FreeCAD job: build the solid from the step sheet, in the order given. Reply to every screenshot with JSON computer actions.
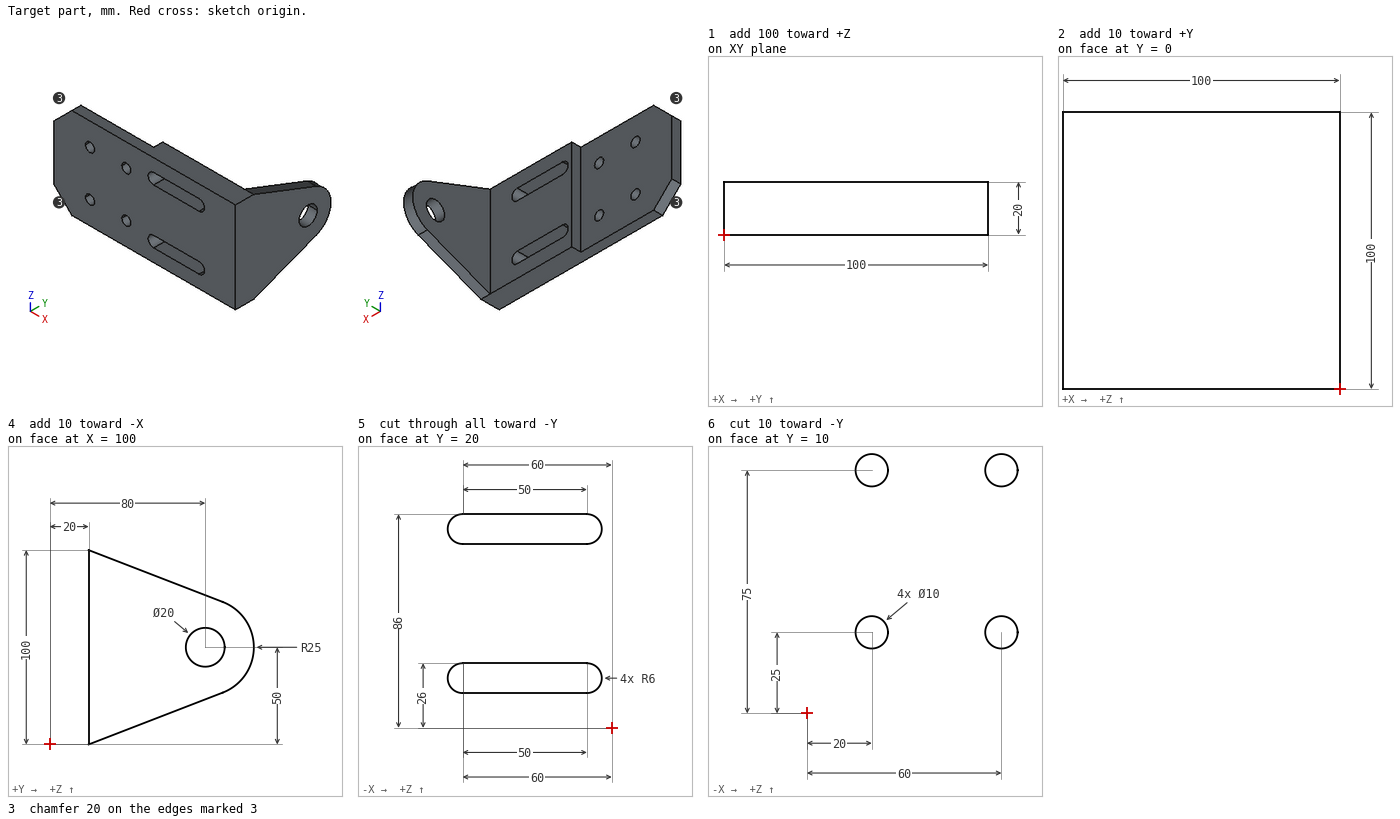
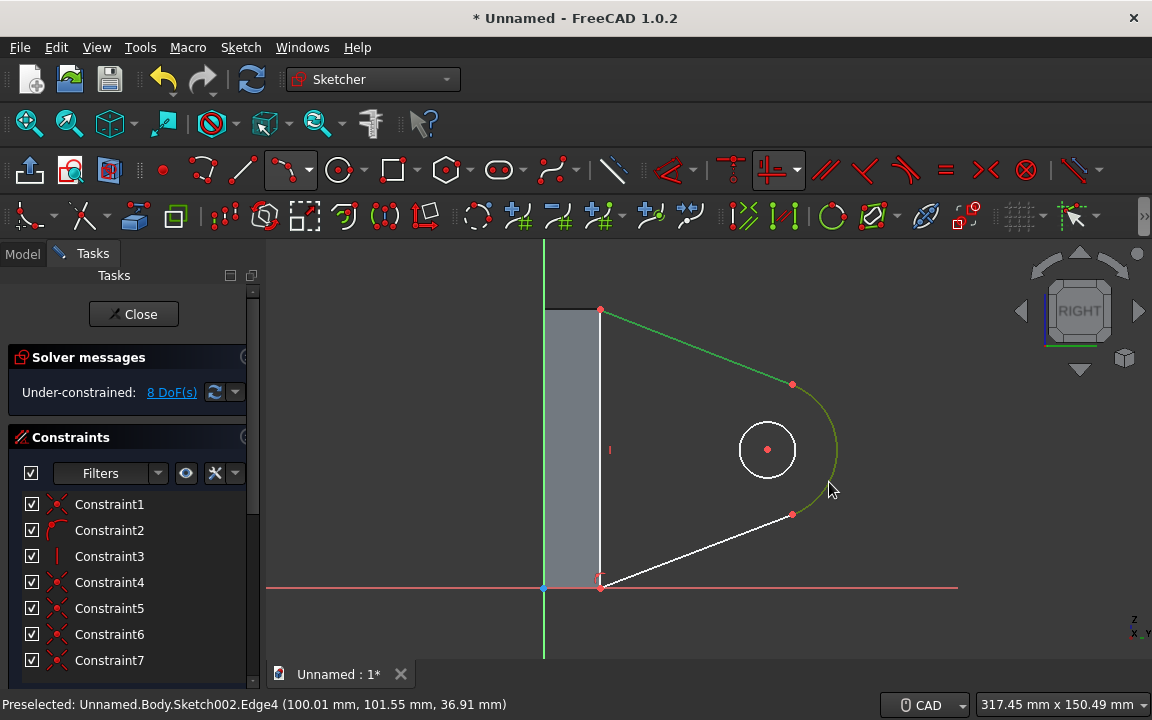
{"action": "left_click", "coordinate": [906, 170]}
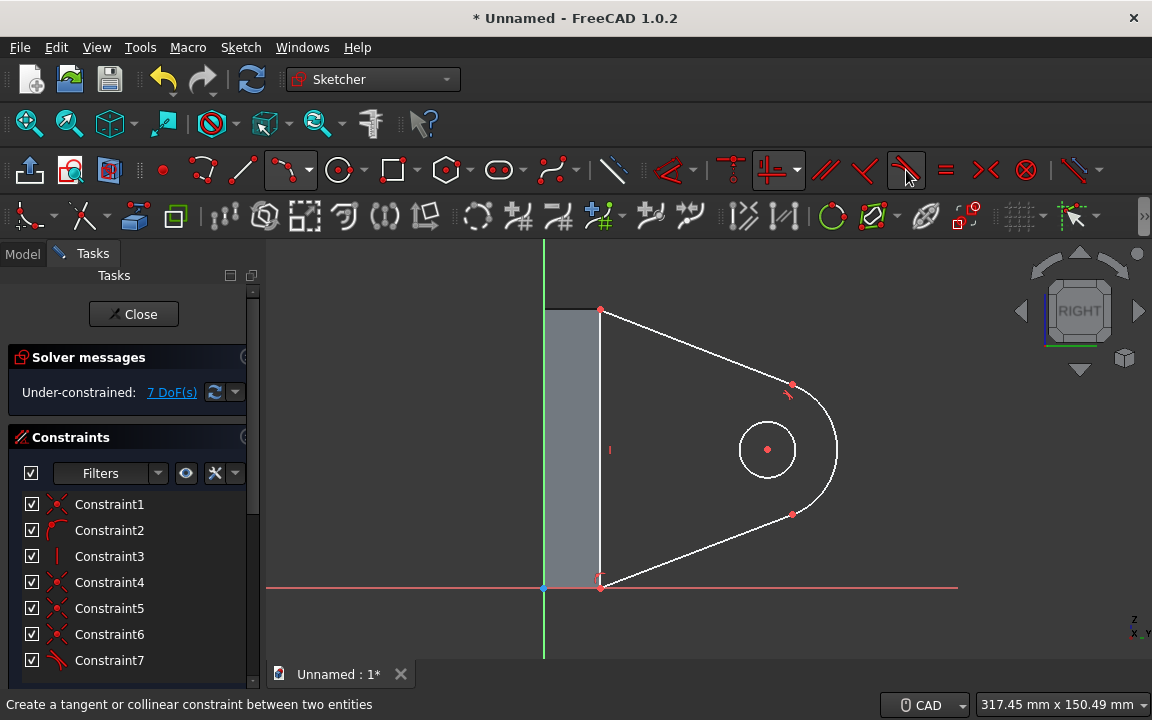
{"action": "left_click", "coordinate": [658, 566]}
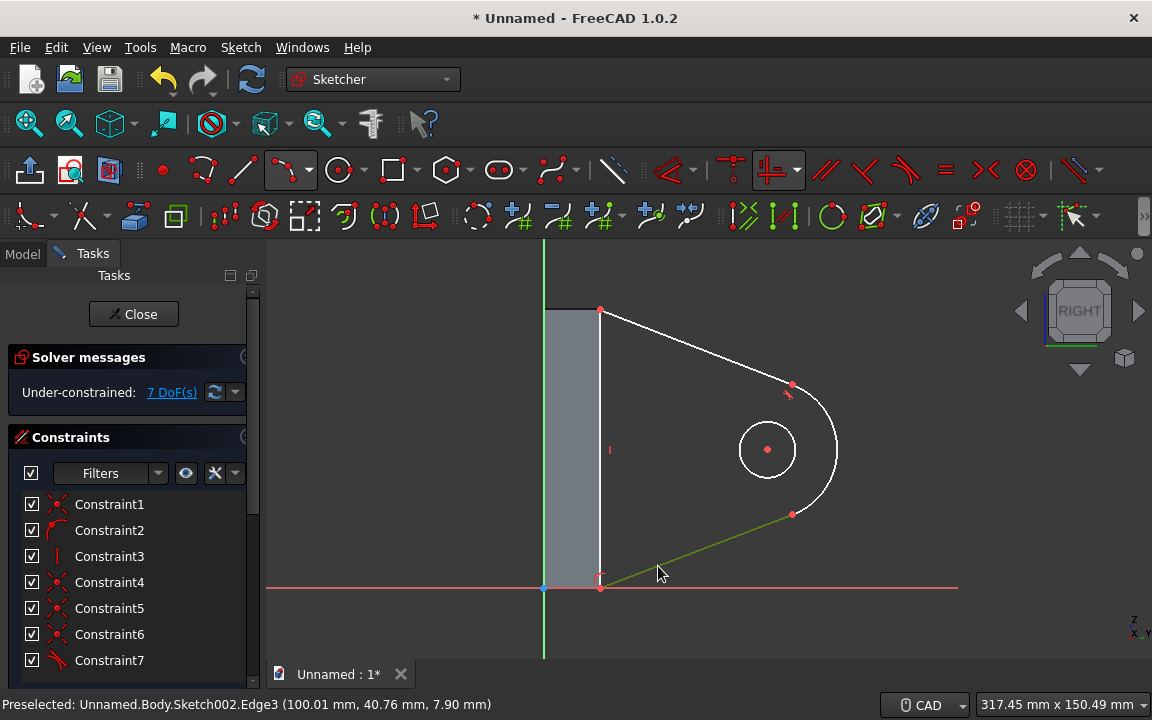
{"action": "left_click", "coordinate": [829, 482]}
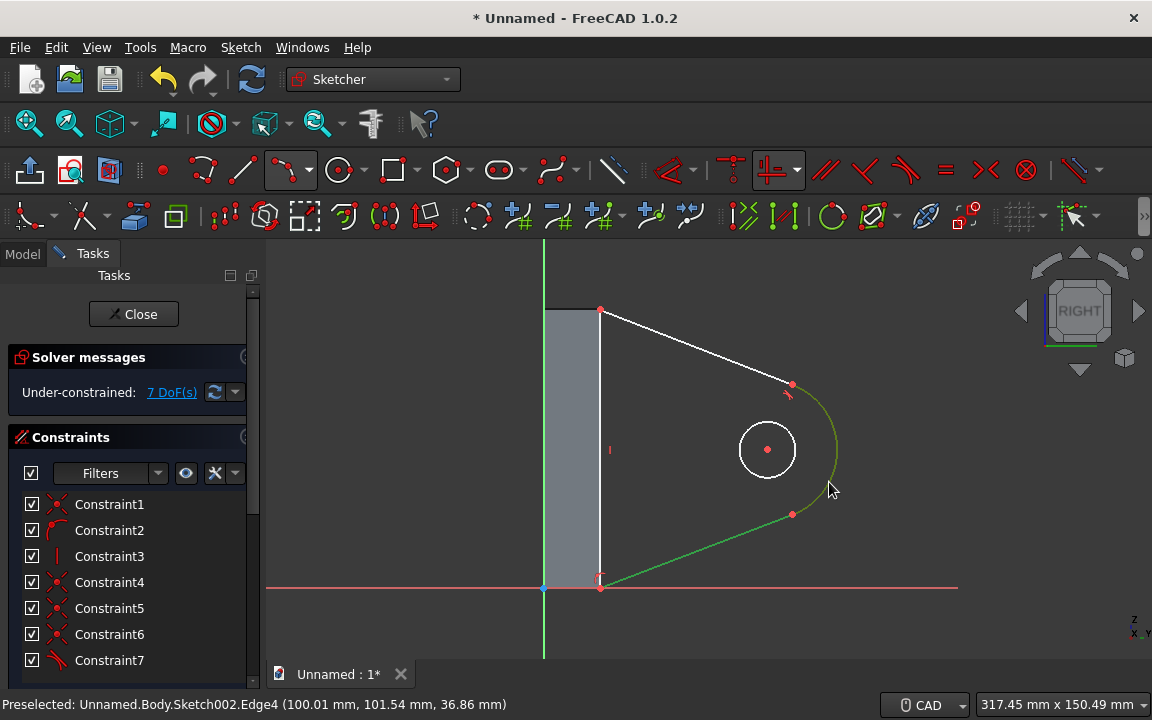
{"action": "left_click", "coordinate": [906, 170]}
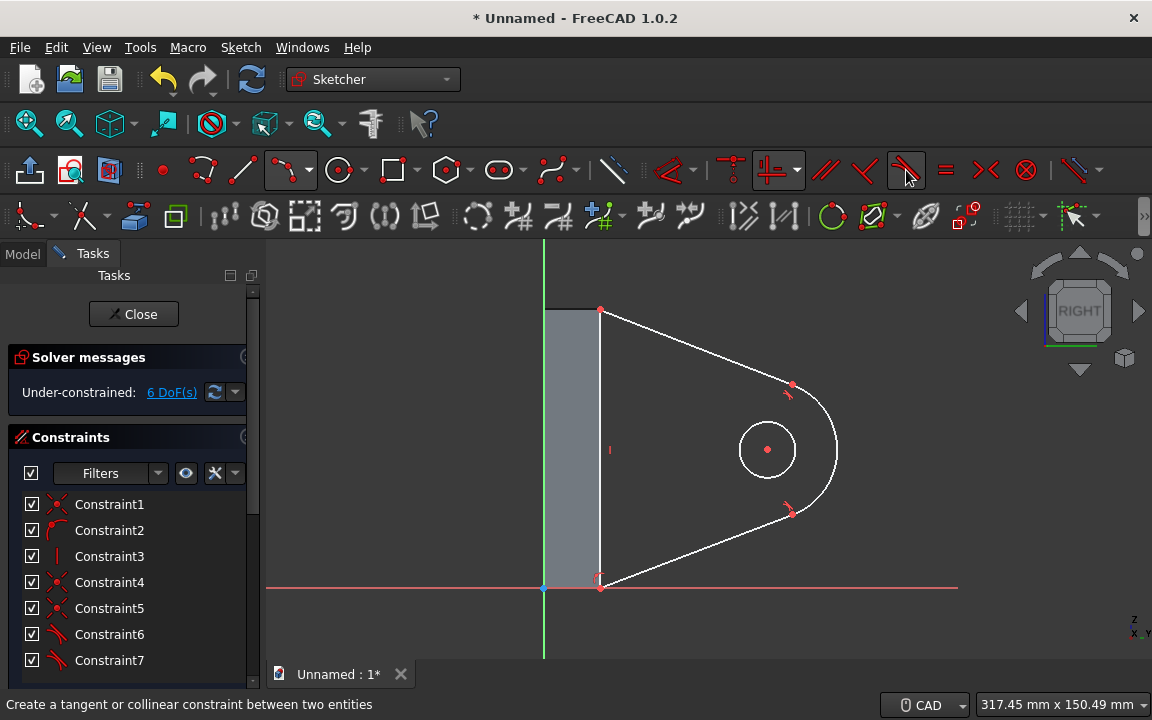
{"action": "left_click", "coordinate": [668, 170]}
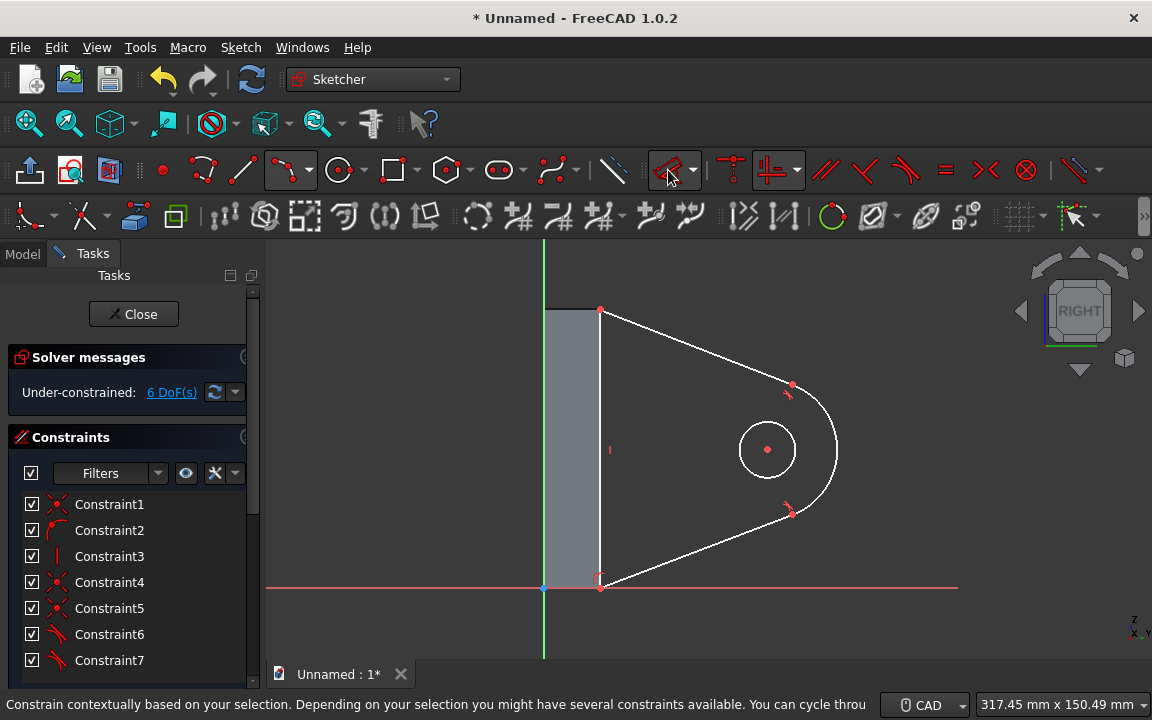
{"action": "left_click", "coordinate": [829, 482]}
{"action": "left_click", "coordinate": [857, 497]}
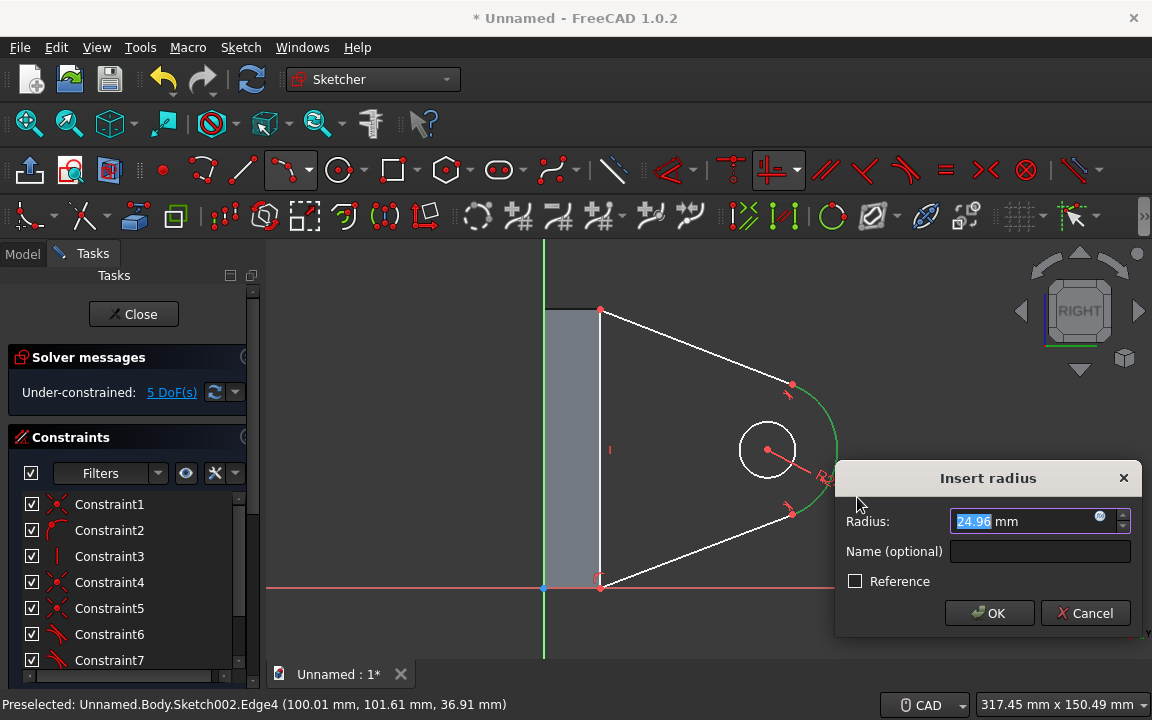
{"action": "type", "text": "25"}
{"action": "key", "text": "Return"}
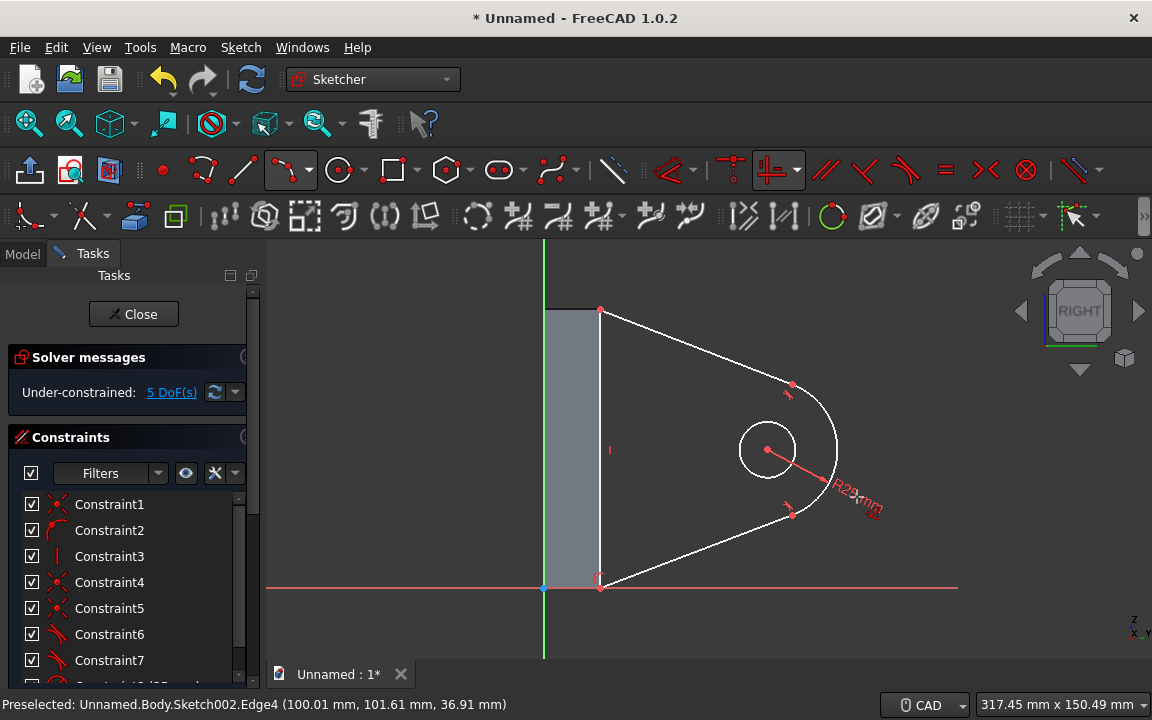
{"action": "left_click", "coordinate": [787, 430]}
{"action": "left_click", "coordinate": [754, 392]}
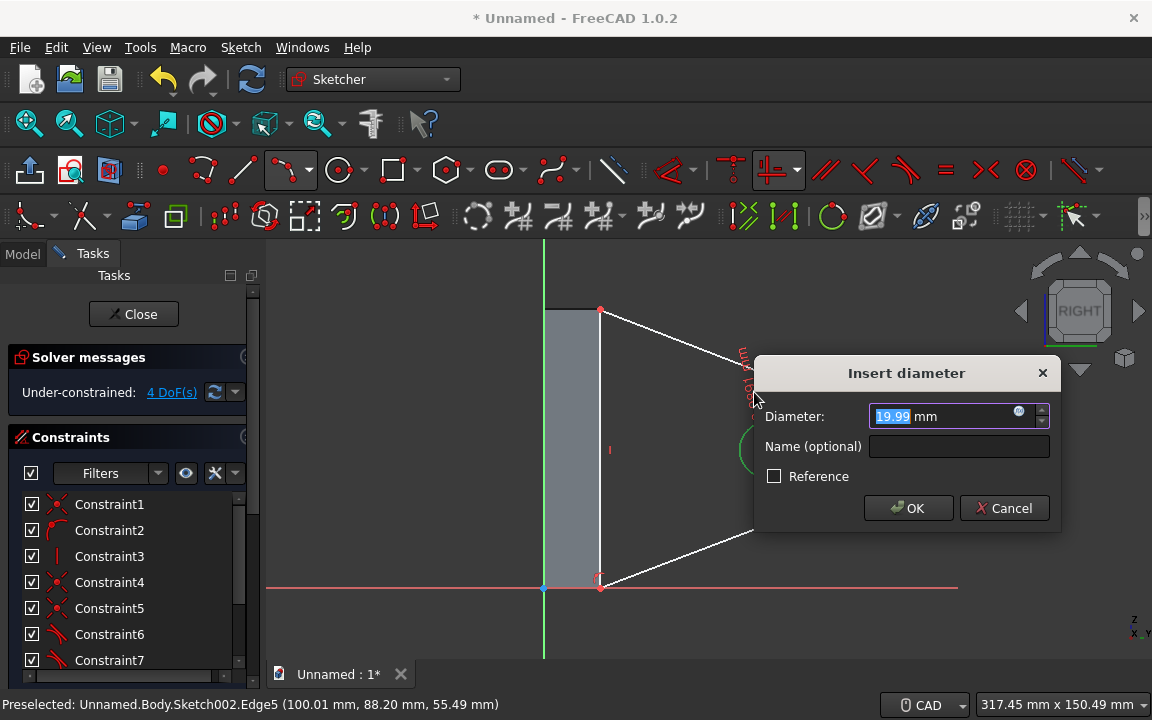
{"action": "type", "text": "20"}
{"action": "key", "text": "Return"}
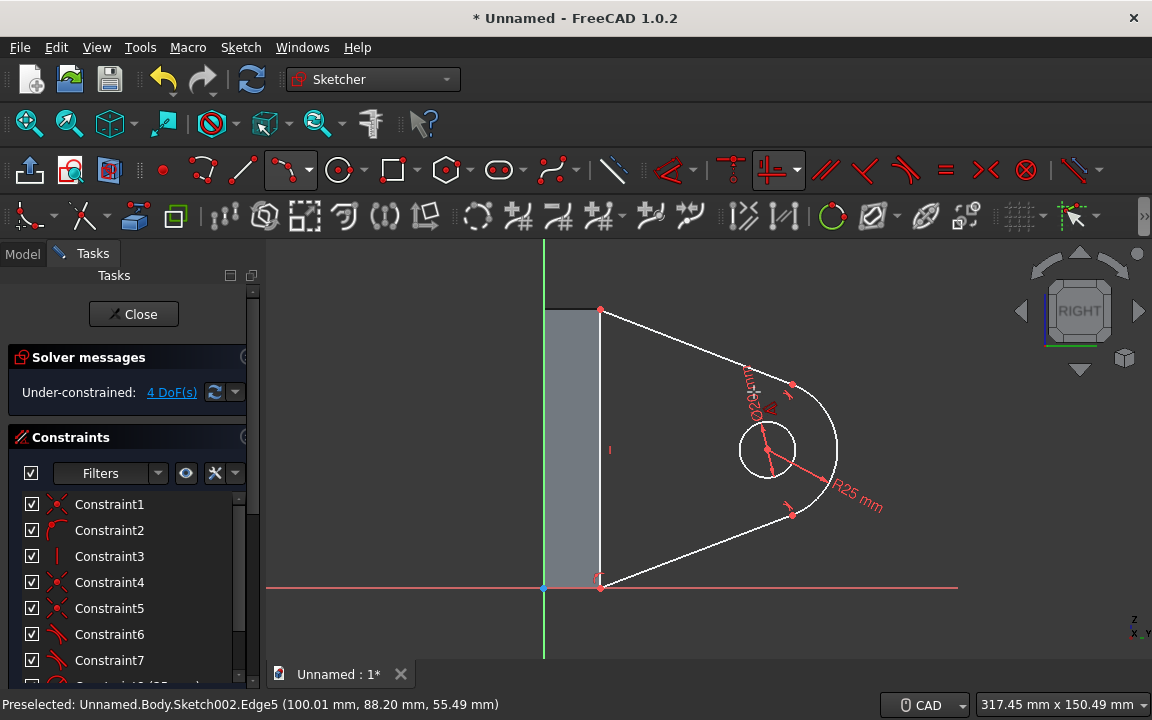
{"action": "left_click", "coordinate": [768, 450]}
{"action": "left_click", "coordinate": [656, 622]}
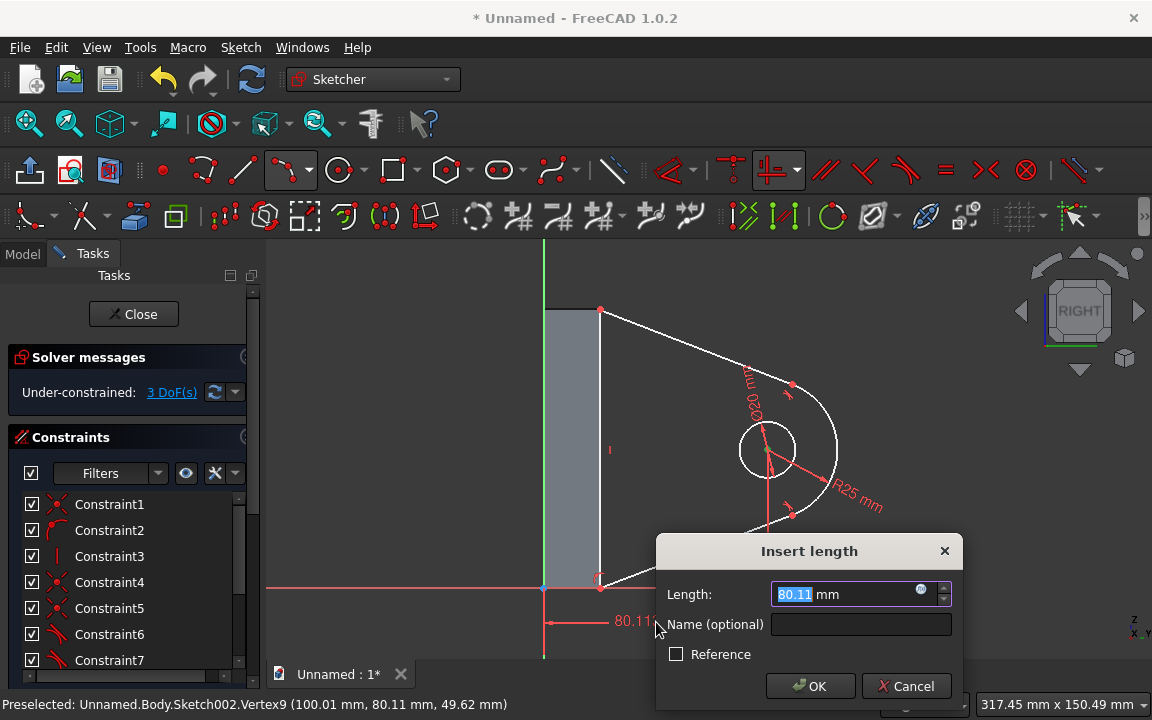
{"action": "type", "text": "80"}
{"action": "key", "text": "Return"}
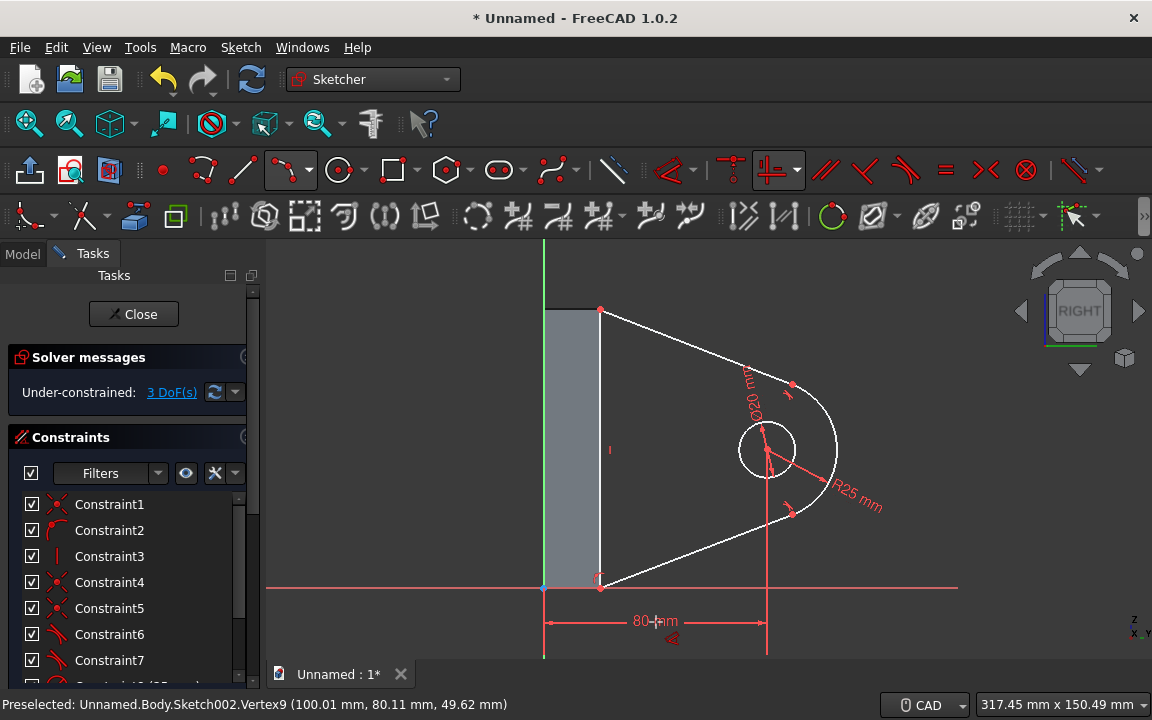
{"action": "left_click", "coordinate": [767, 450]}
{"action": "left_click", "coordinate": [510, 519]}